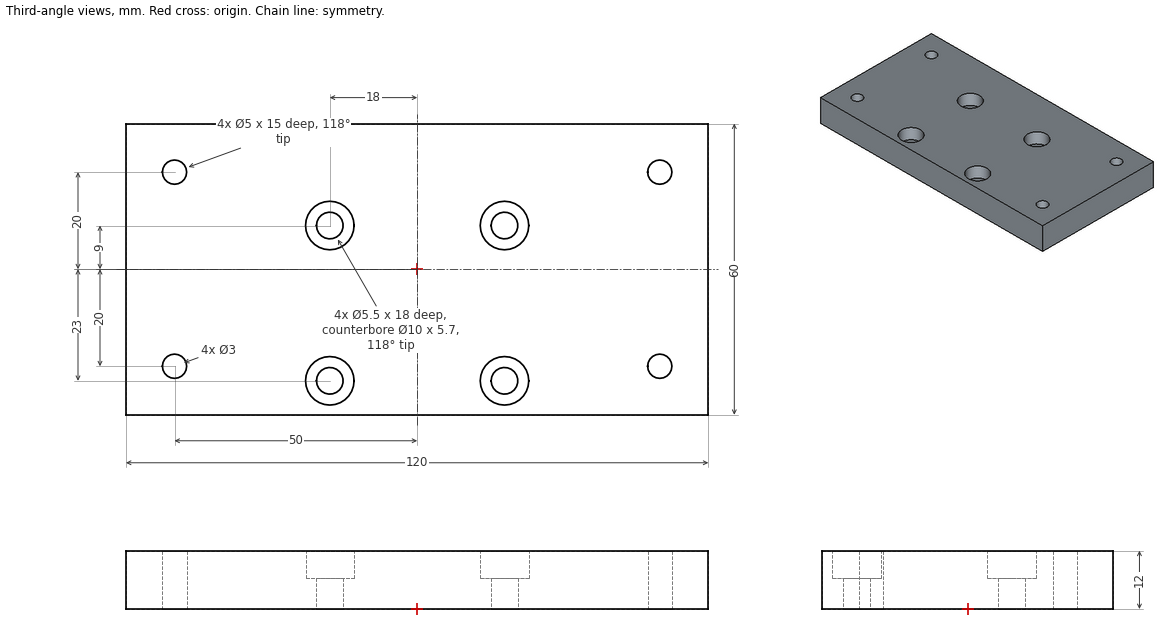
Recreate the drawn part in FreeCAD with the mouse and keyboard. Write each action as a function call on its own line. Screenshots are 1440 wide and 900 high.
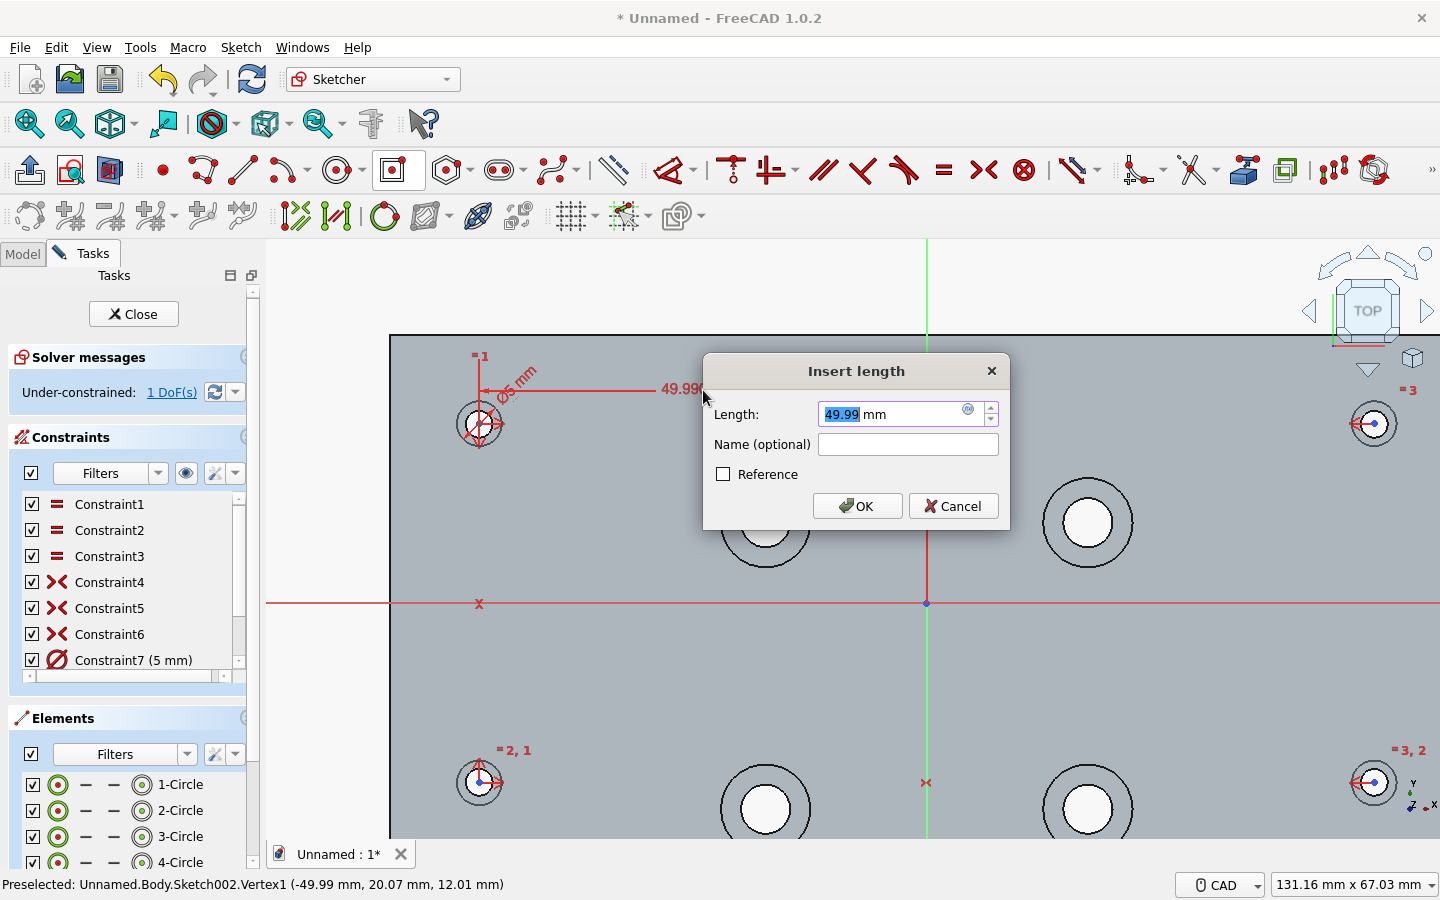
text(50)
key(Return)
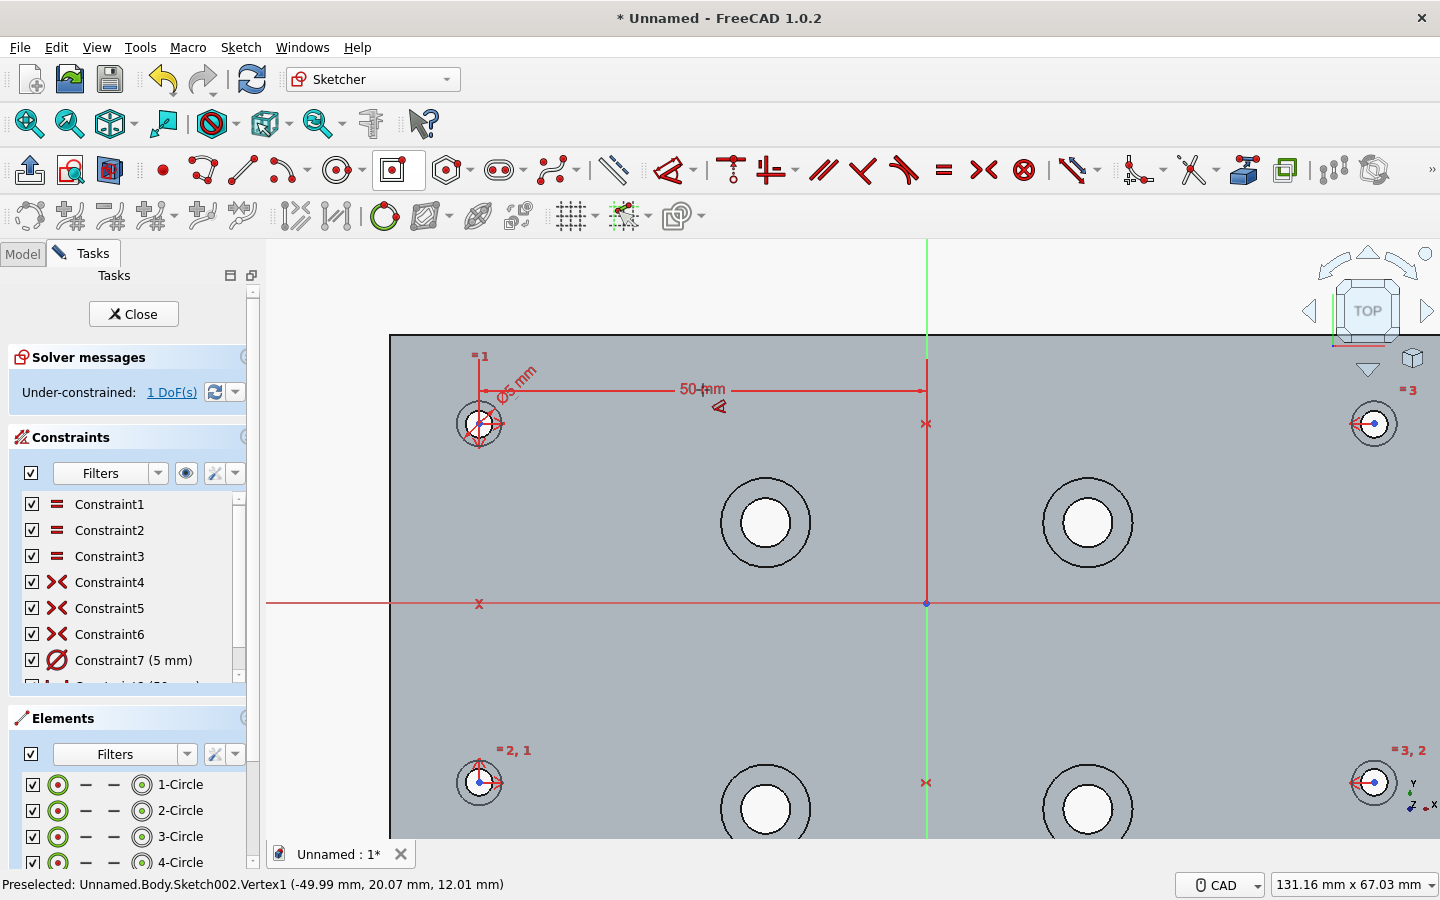
click(479, 424)
click(445, 513)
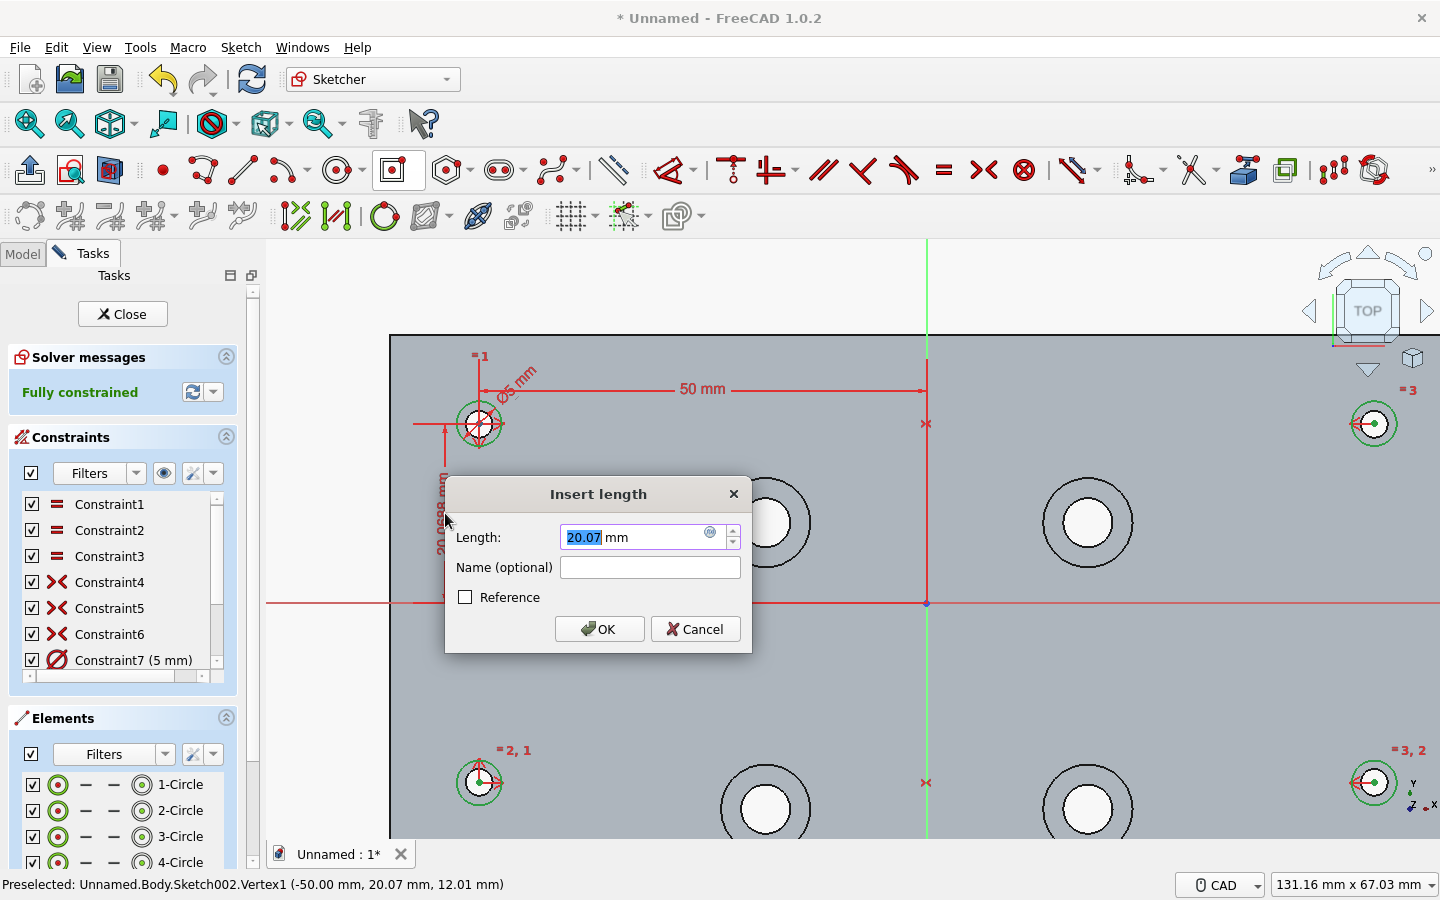
text(20)
key(Return)
key(Escape)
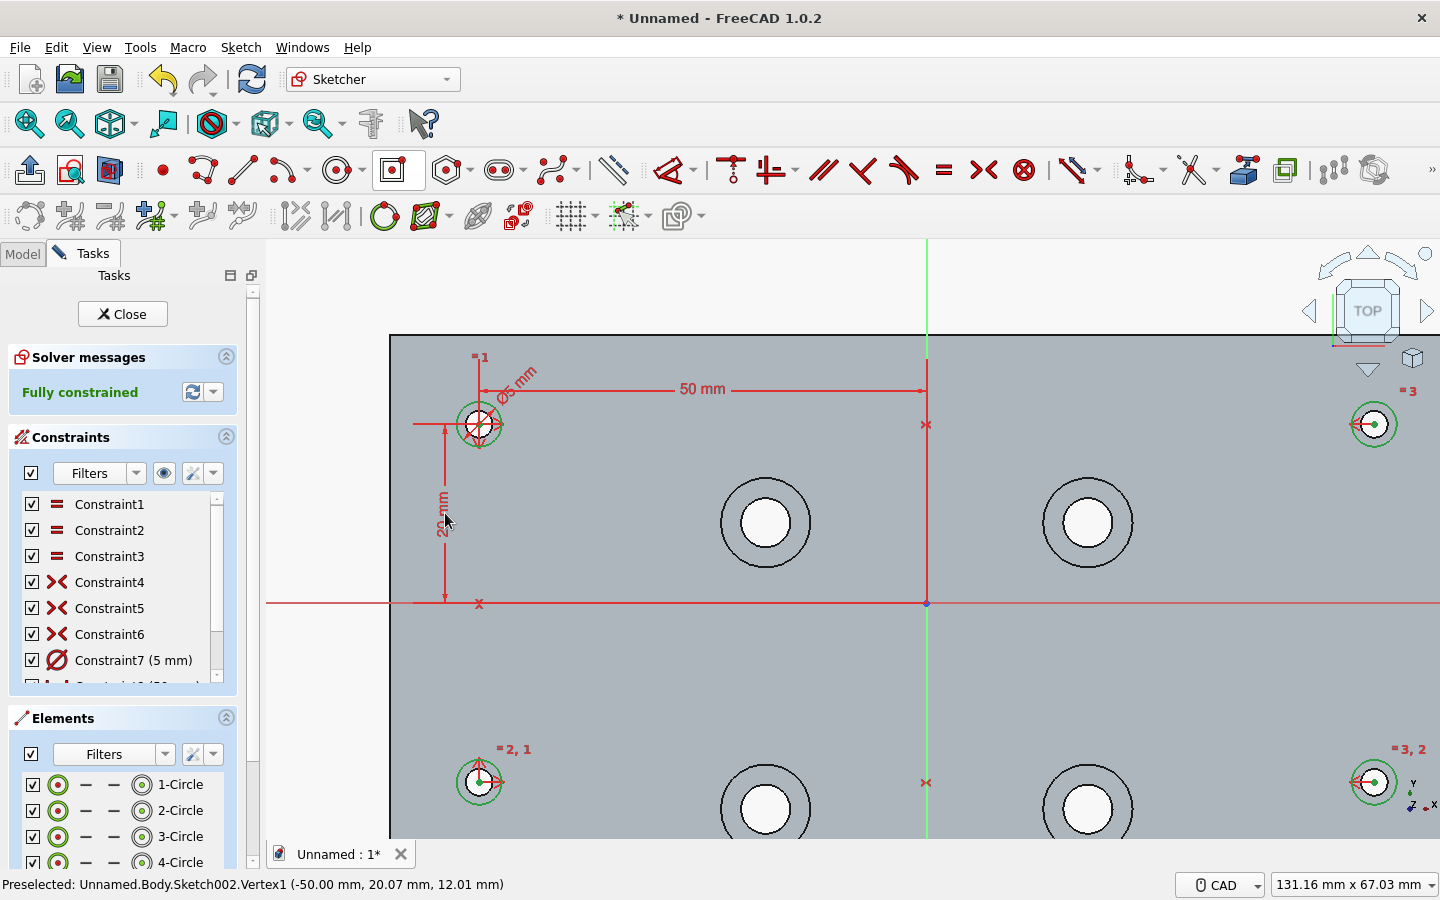
click(123, 314)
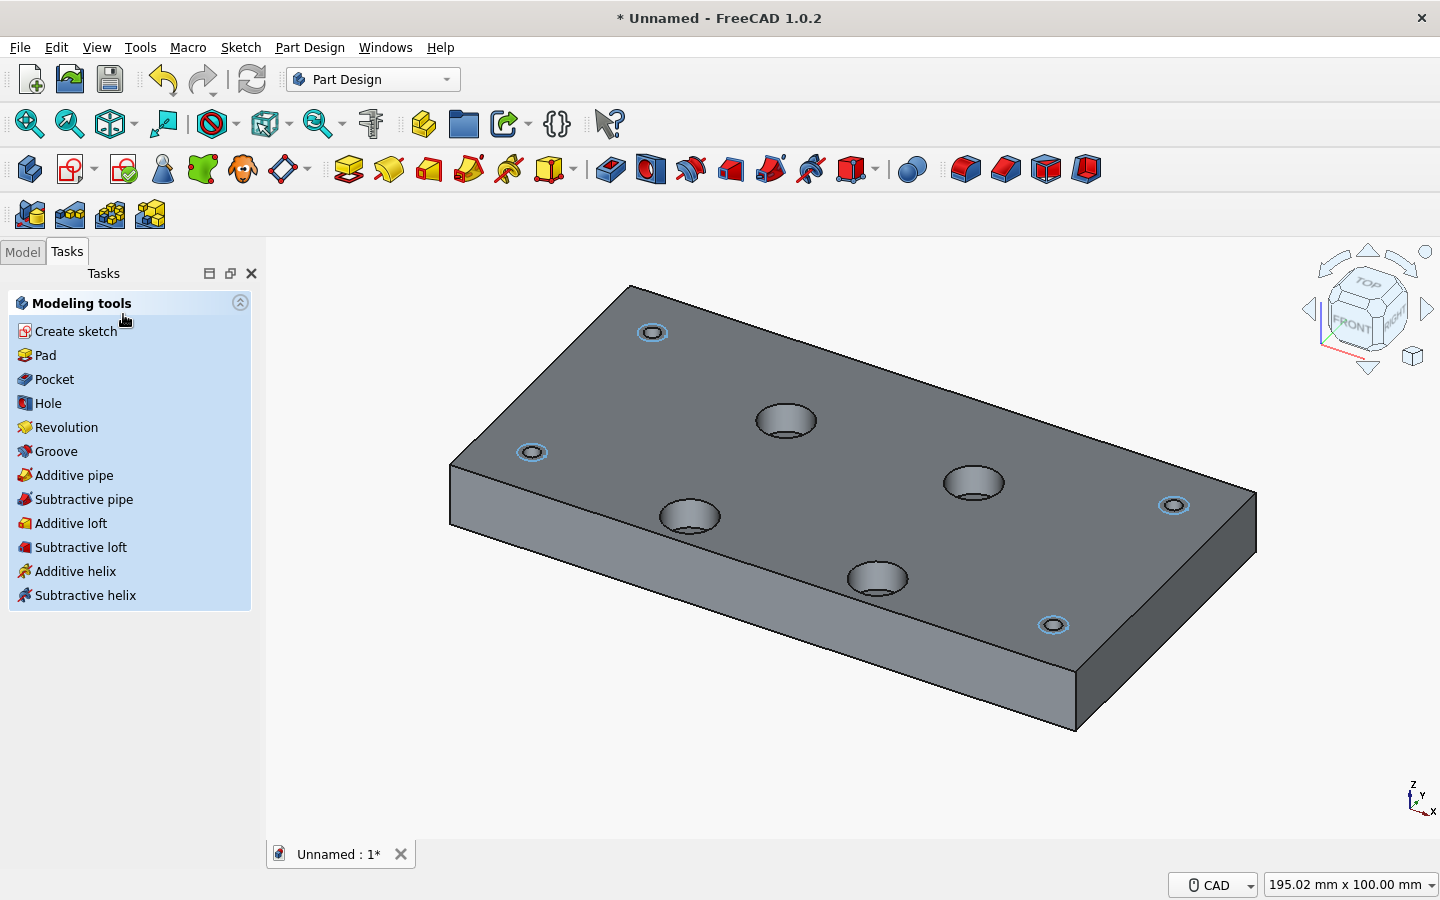
click(652, 170)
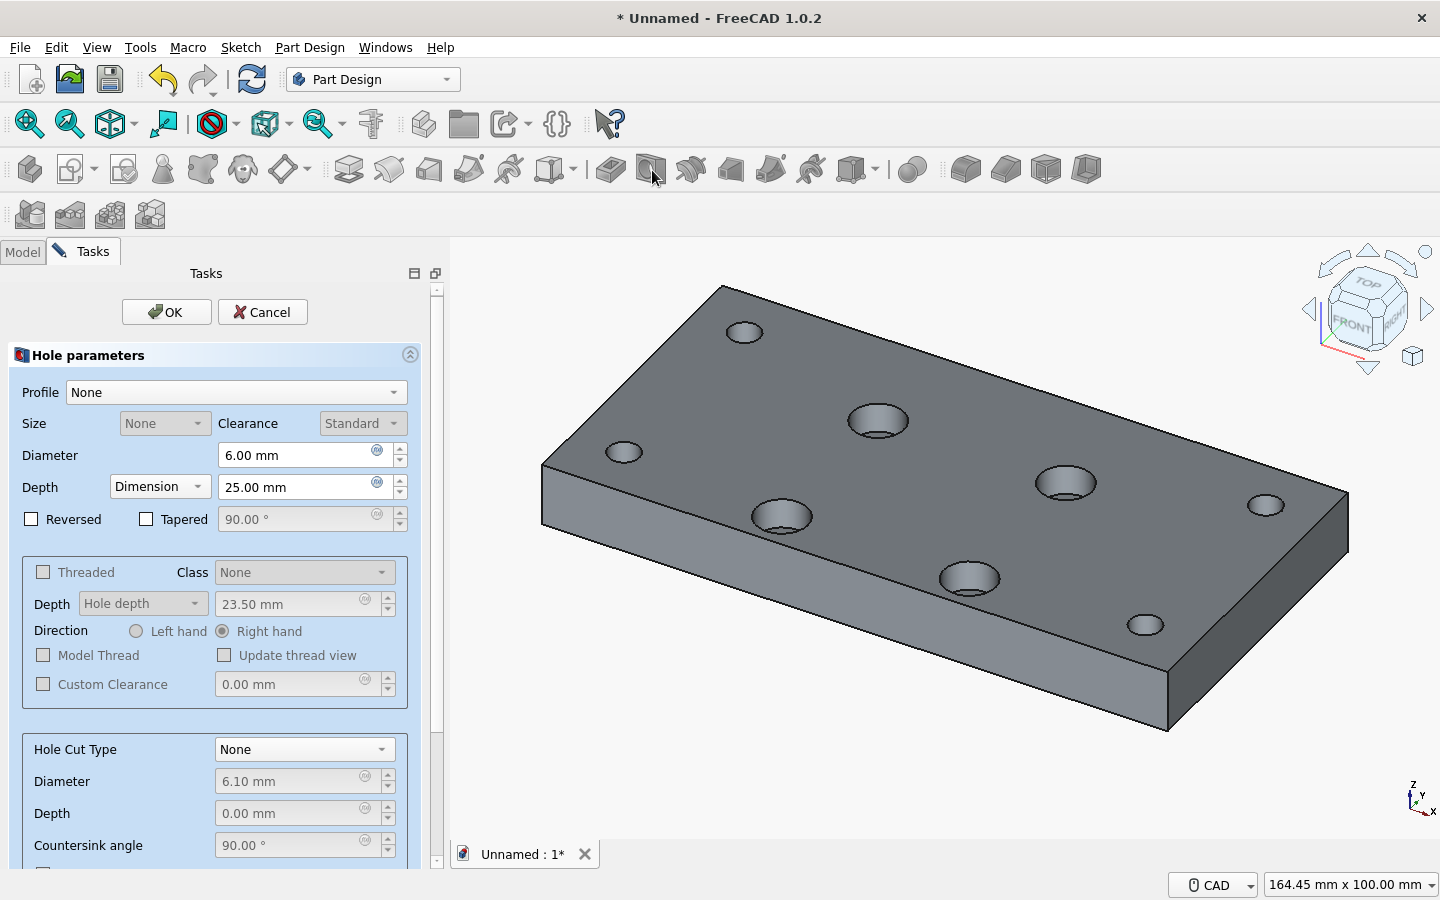
triple_click(305, 455)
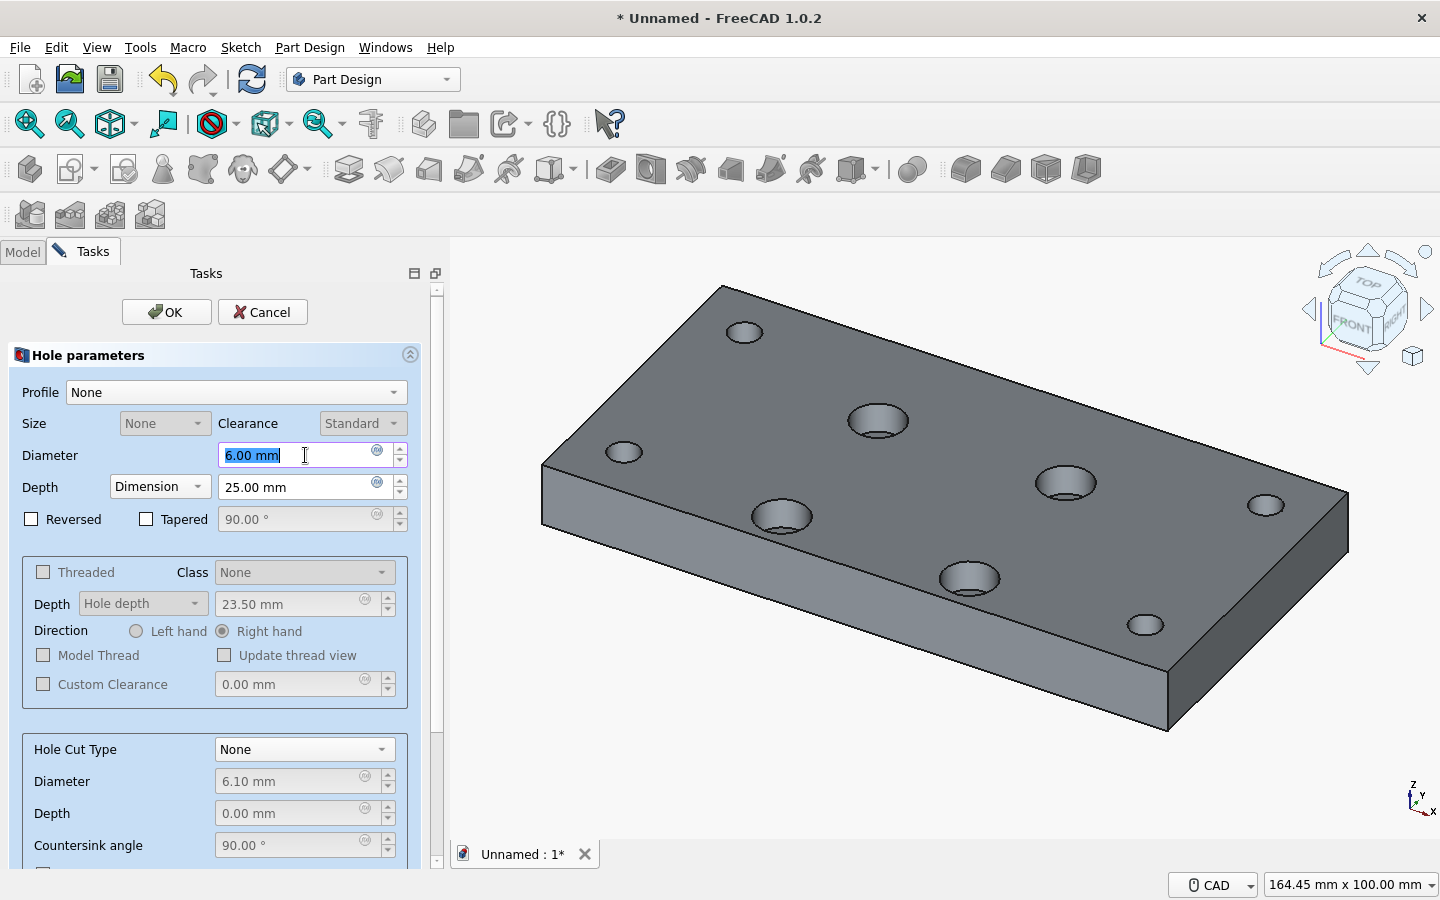
text(5)
key(Tab)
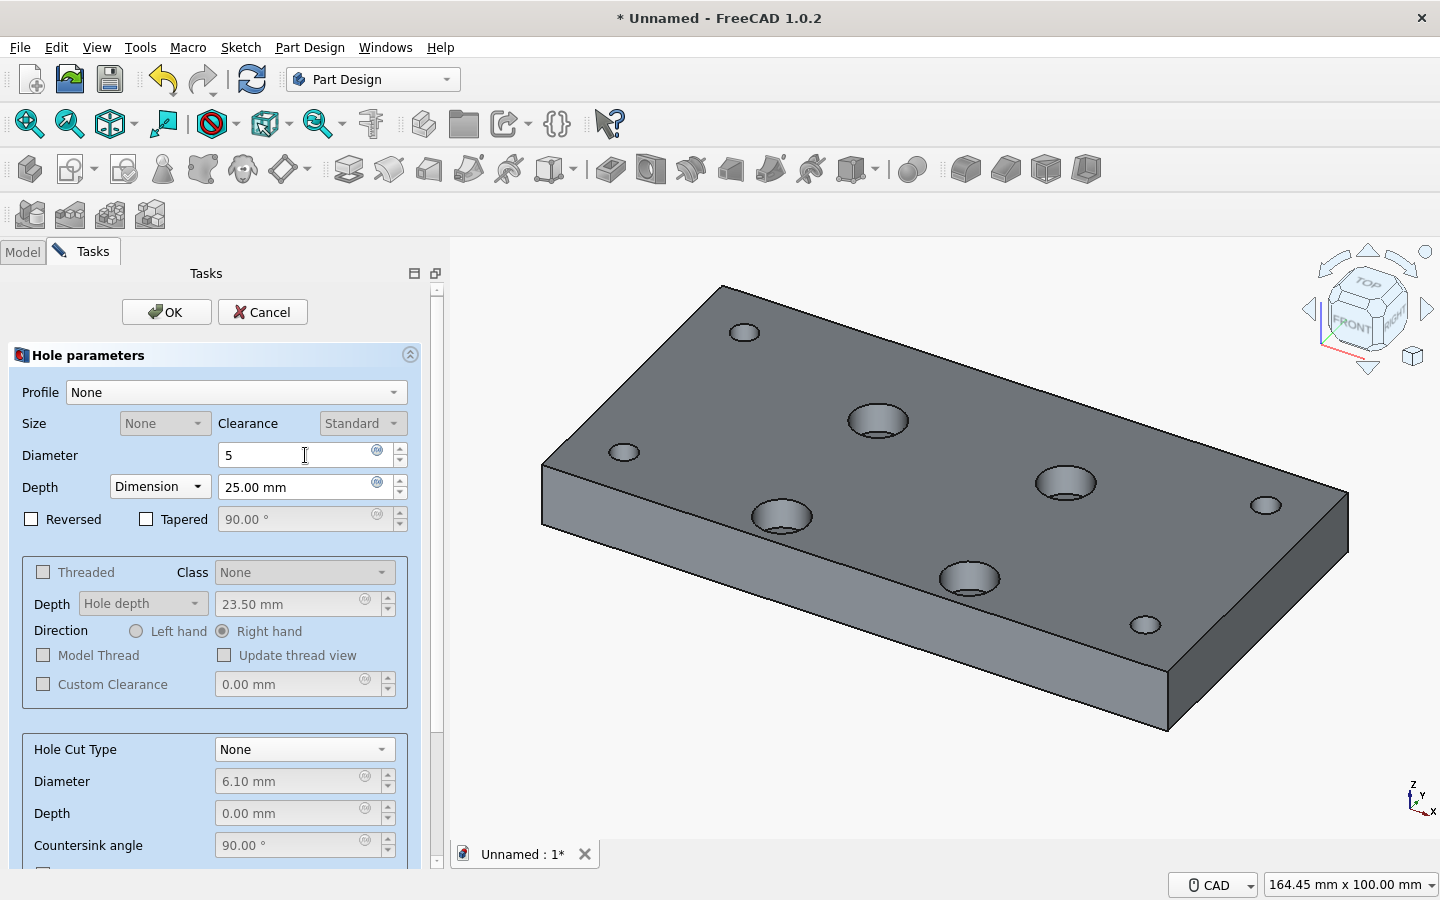
triple_click(305, 487)